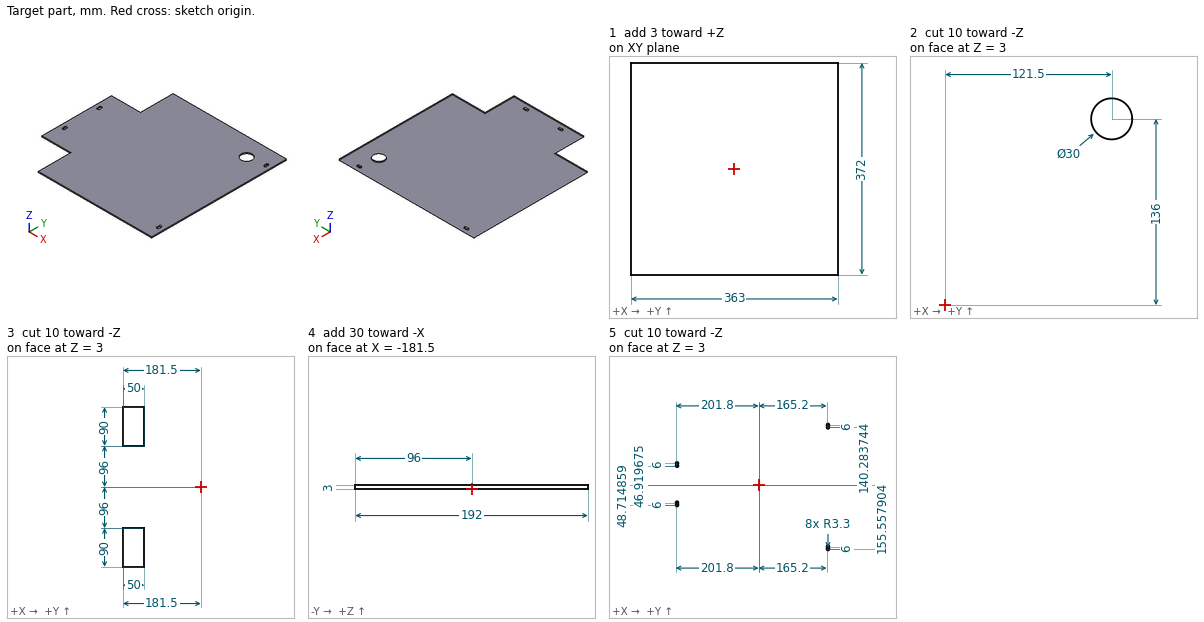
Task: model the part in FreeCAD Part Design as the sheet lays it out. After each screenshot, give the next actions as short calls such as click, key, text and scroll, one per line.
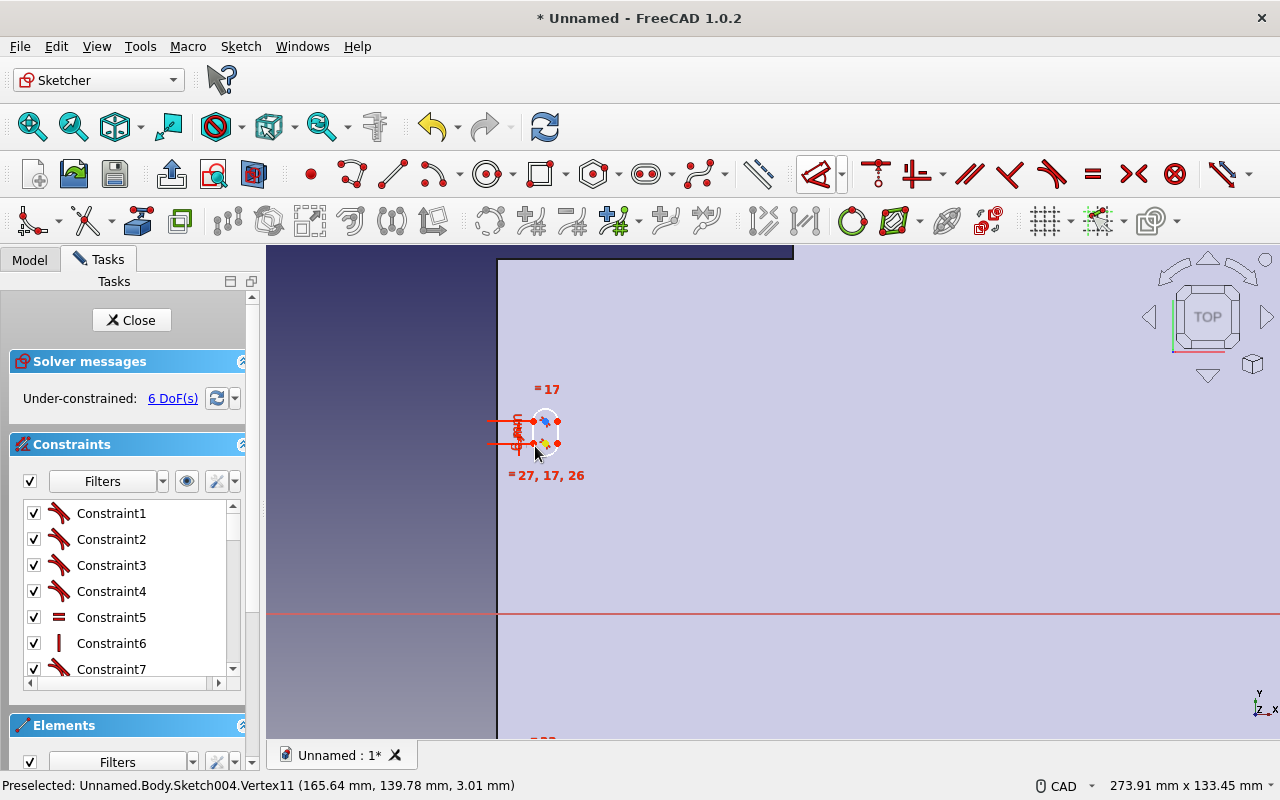
click(533, 444)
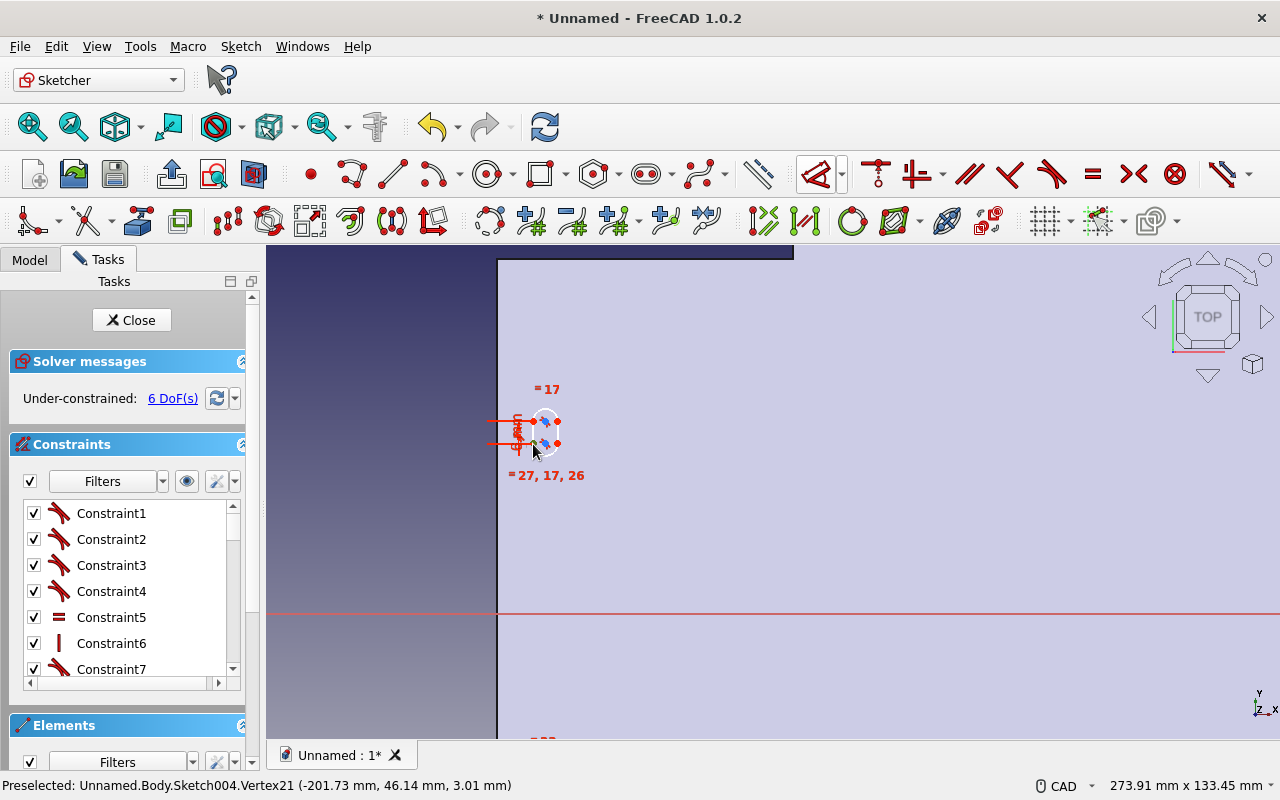
key(l)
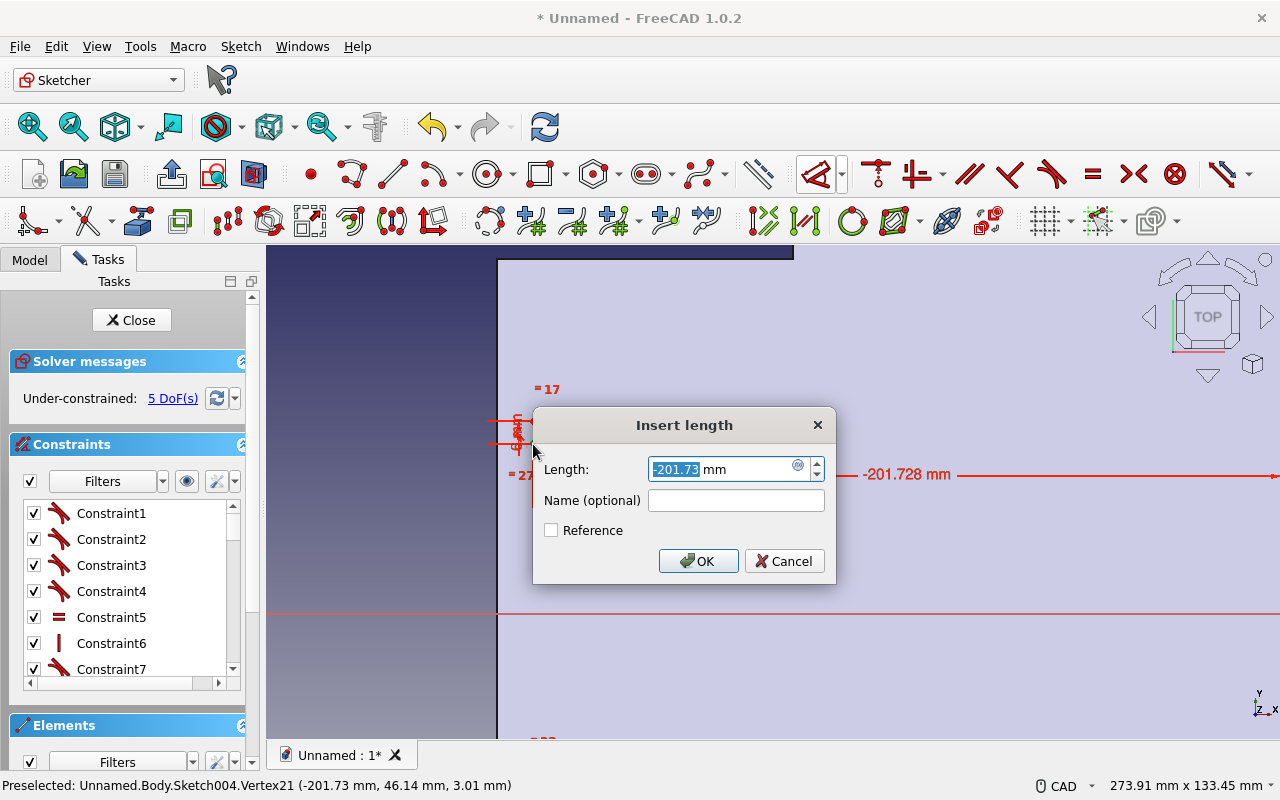
text(-201.8)
key(Return)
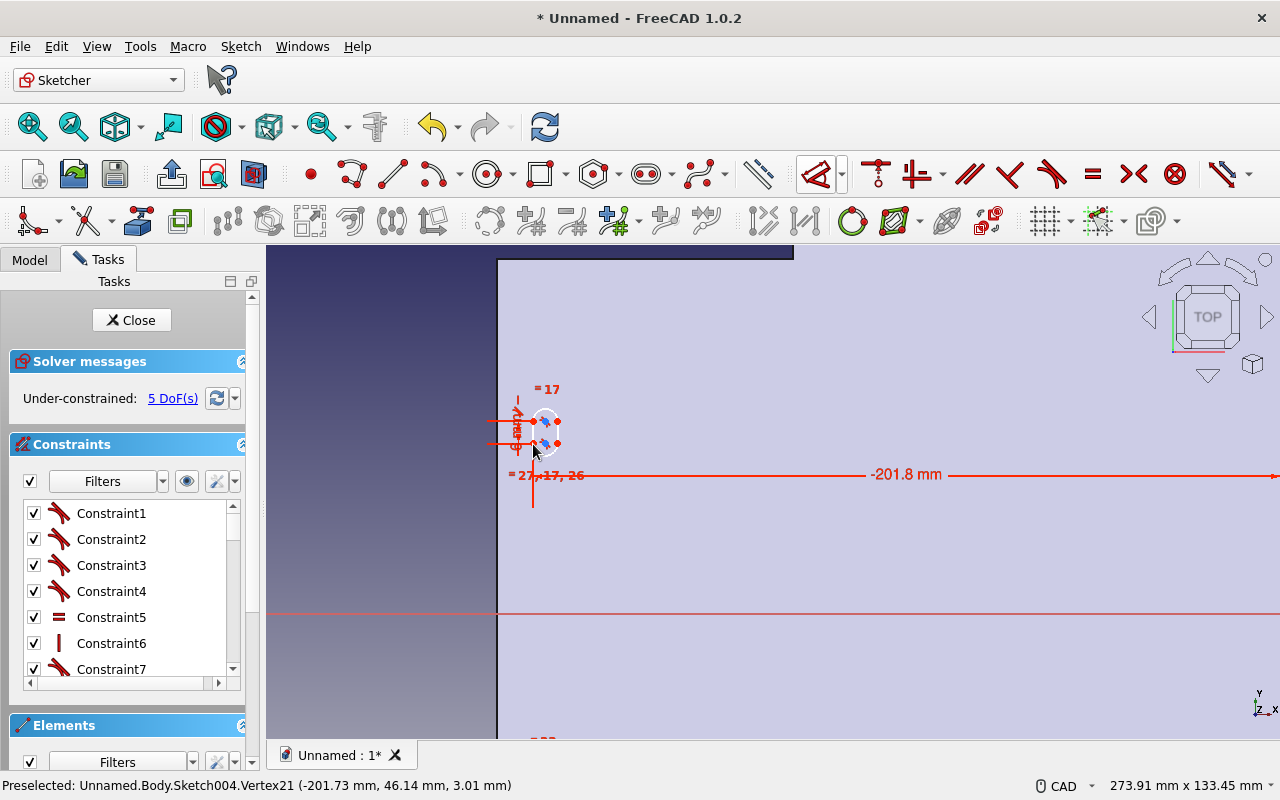
scroll(534, 446, down, 7)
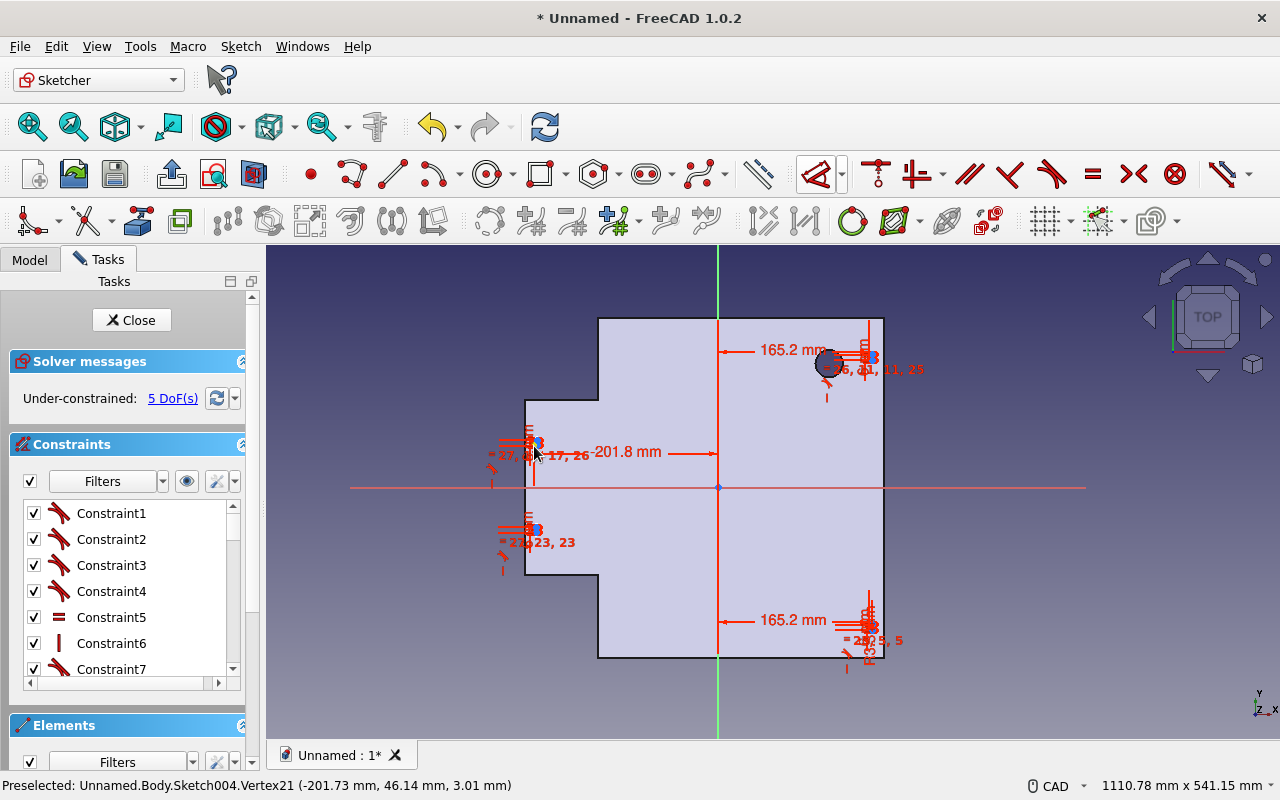
scroll(533, 533, up, 7)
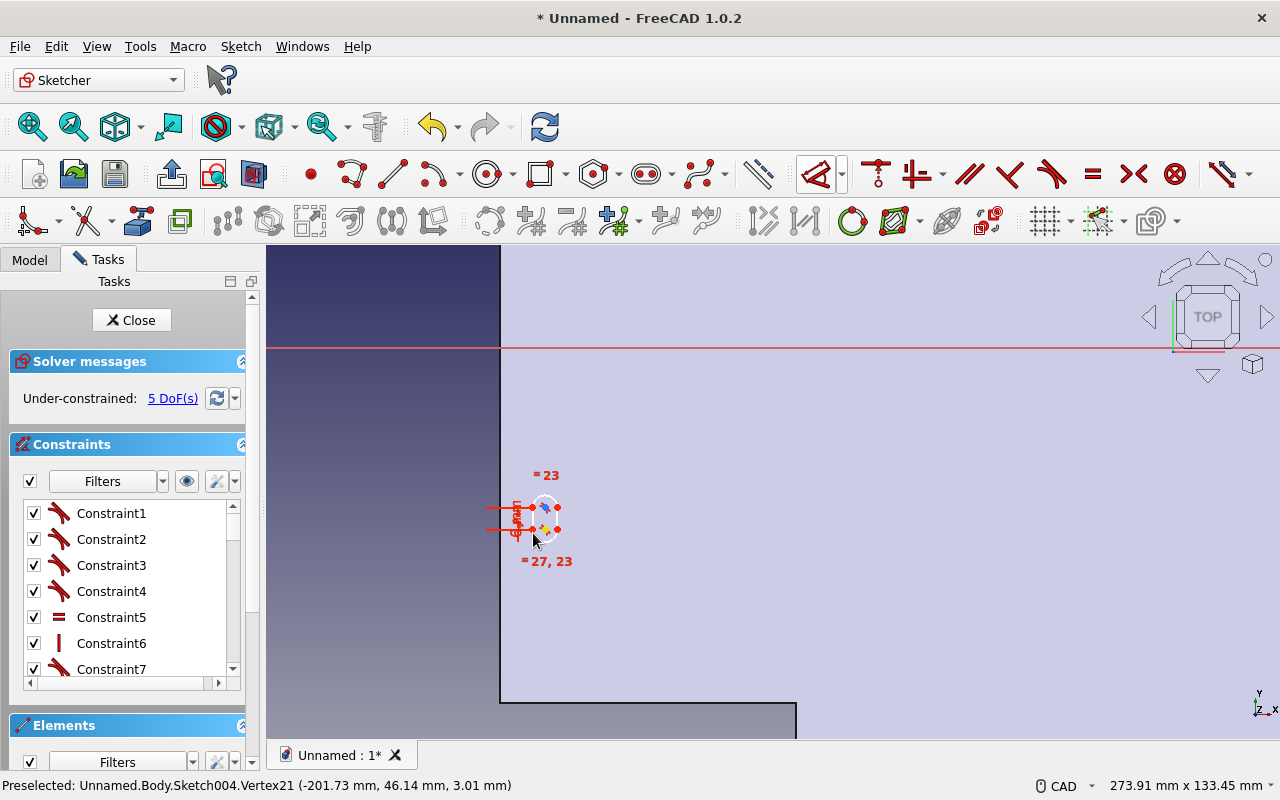
click(533, 530)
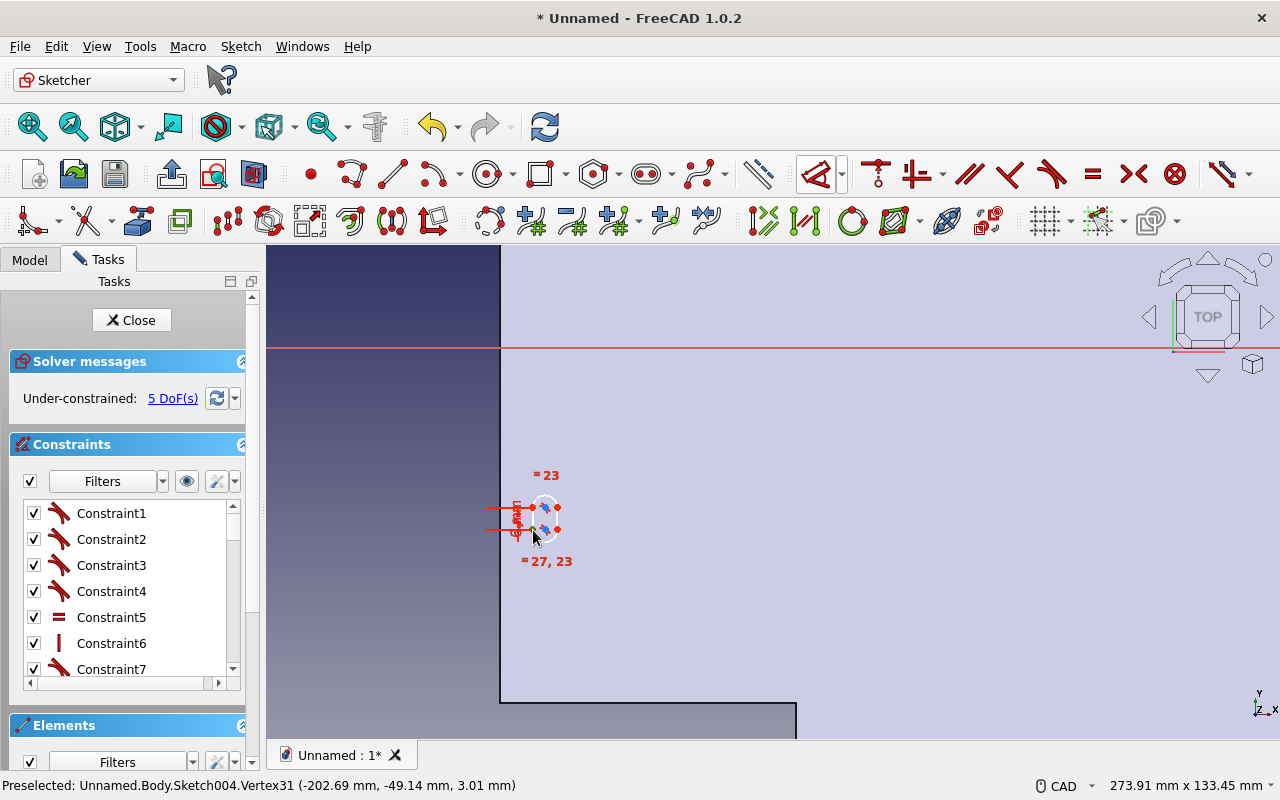
key(l)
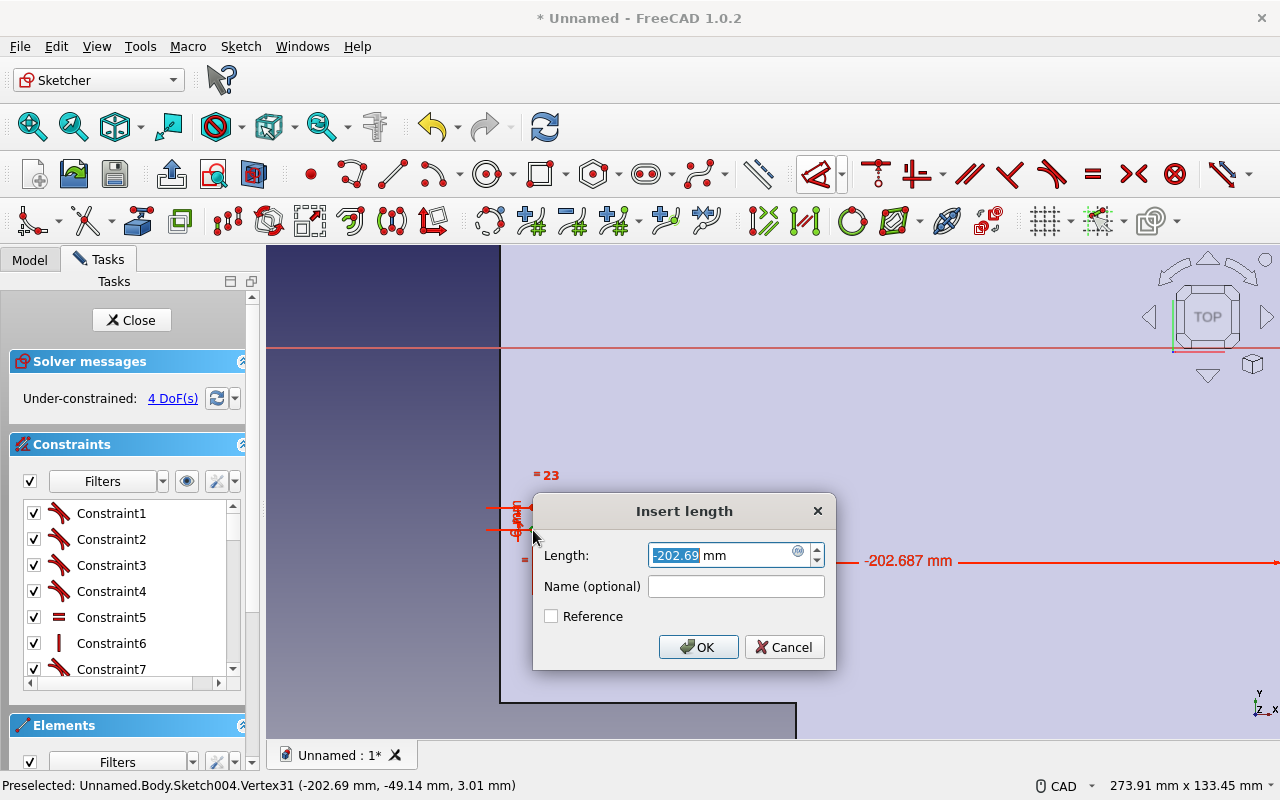
text(-201.8)
key(Return)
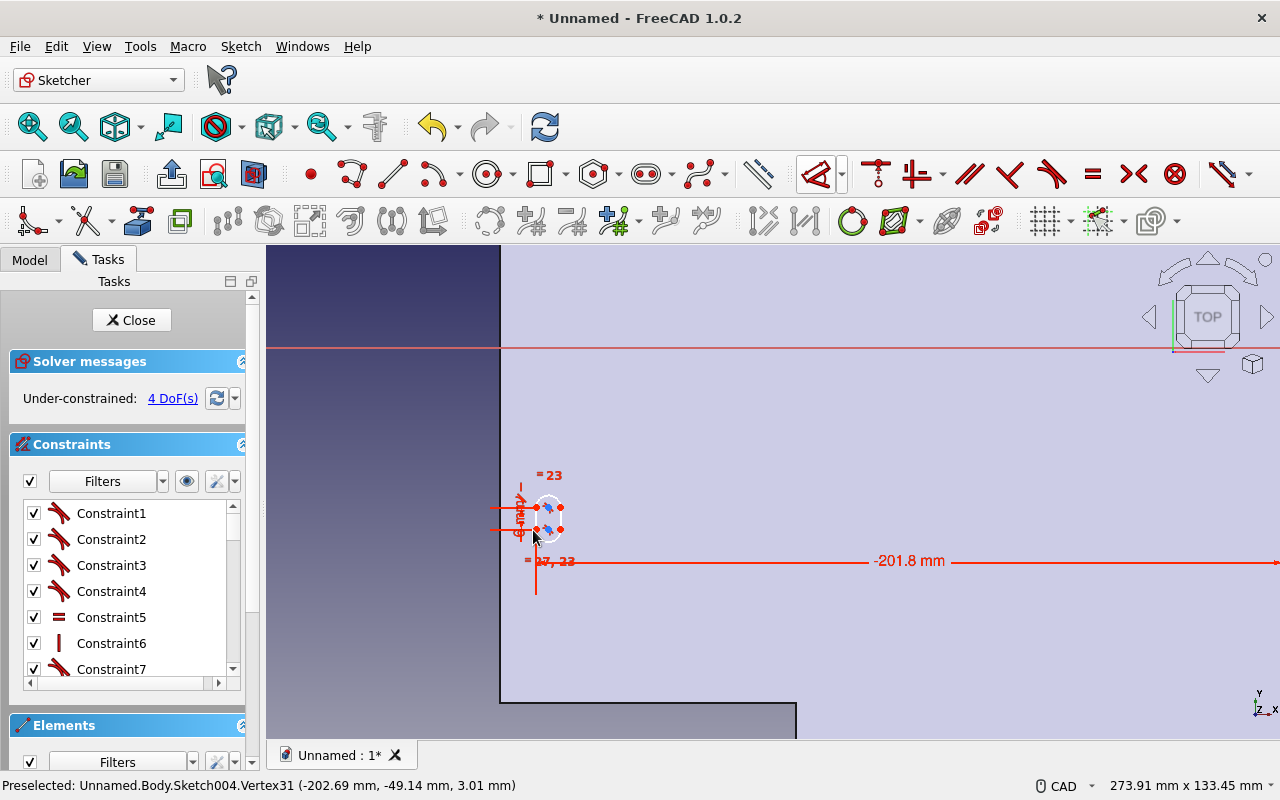
scroll(533, 534, down, 7)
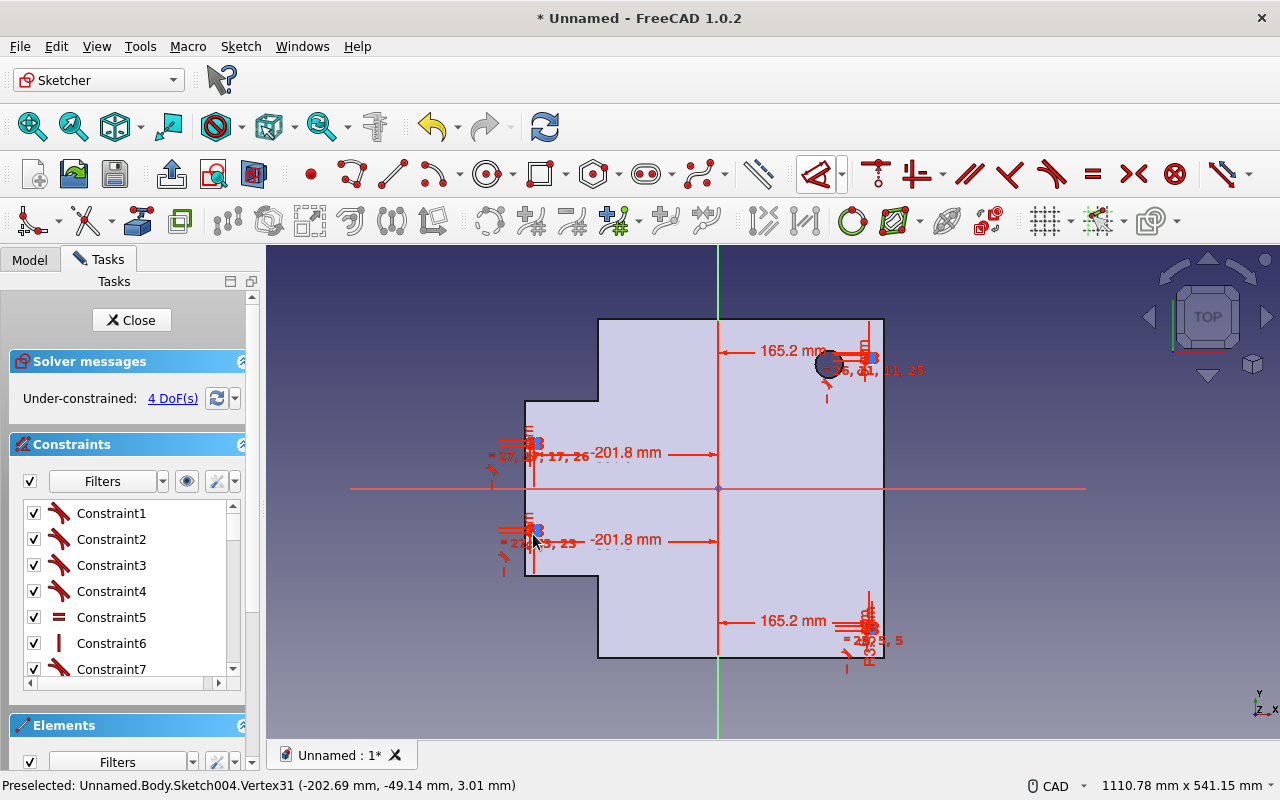
scroll(534, 446, up, 7)